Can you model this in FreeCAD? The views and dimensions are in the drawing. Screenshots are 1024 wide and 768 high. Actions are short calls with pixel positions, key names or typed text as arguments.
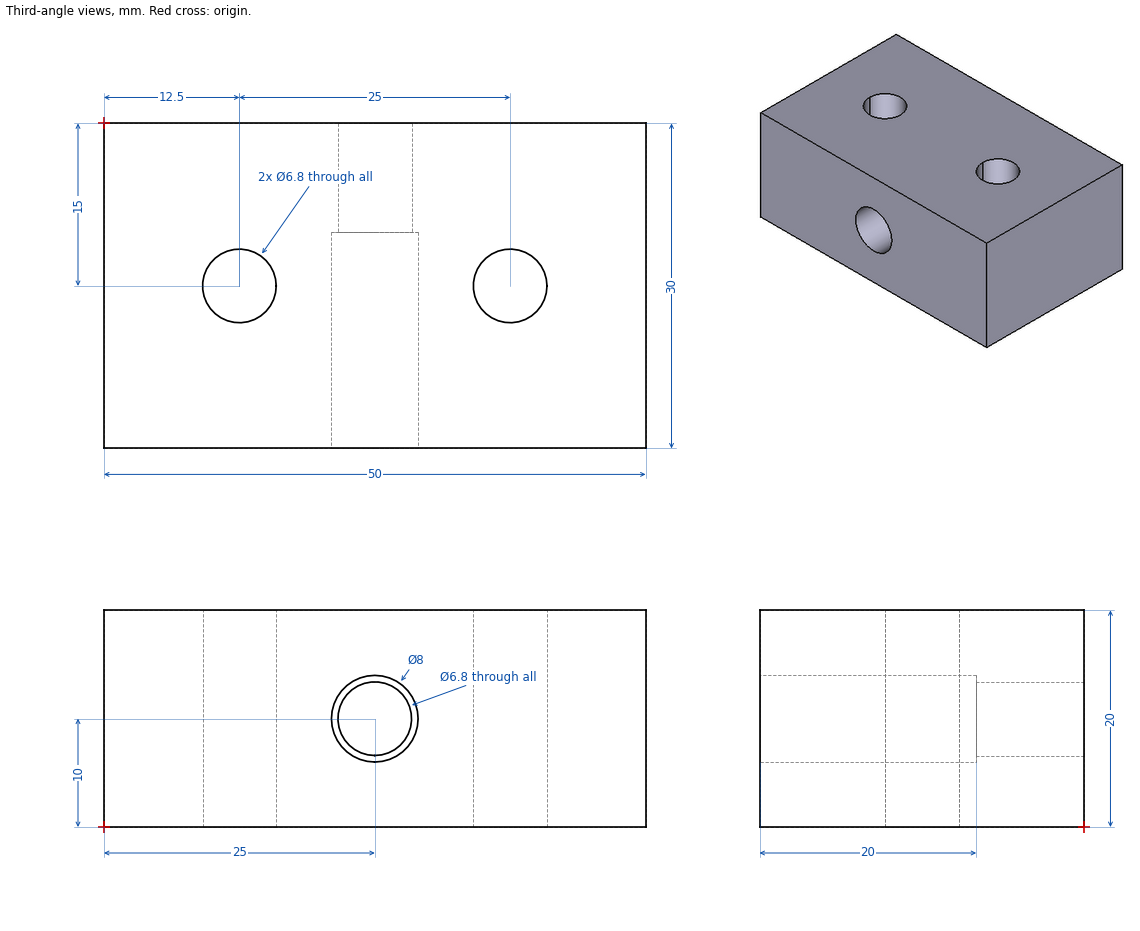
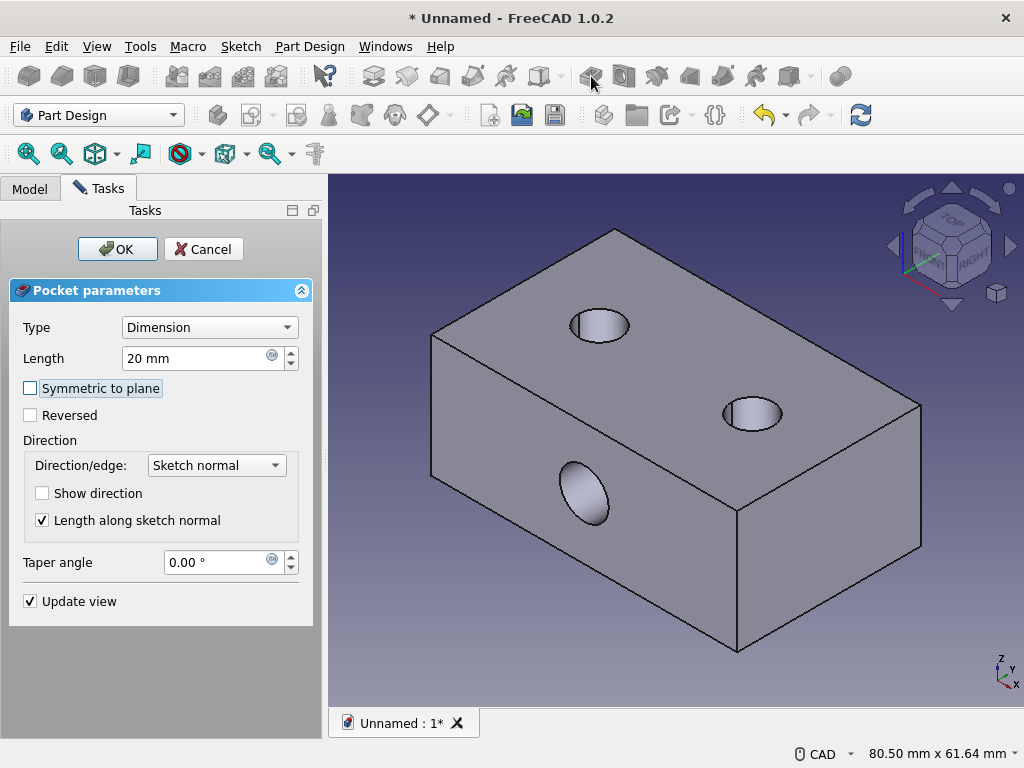
click(118, 249)